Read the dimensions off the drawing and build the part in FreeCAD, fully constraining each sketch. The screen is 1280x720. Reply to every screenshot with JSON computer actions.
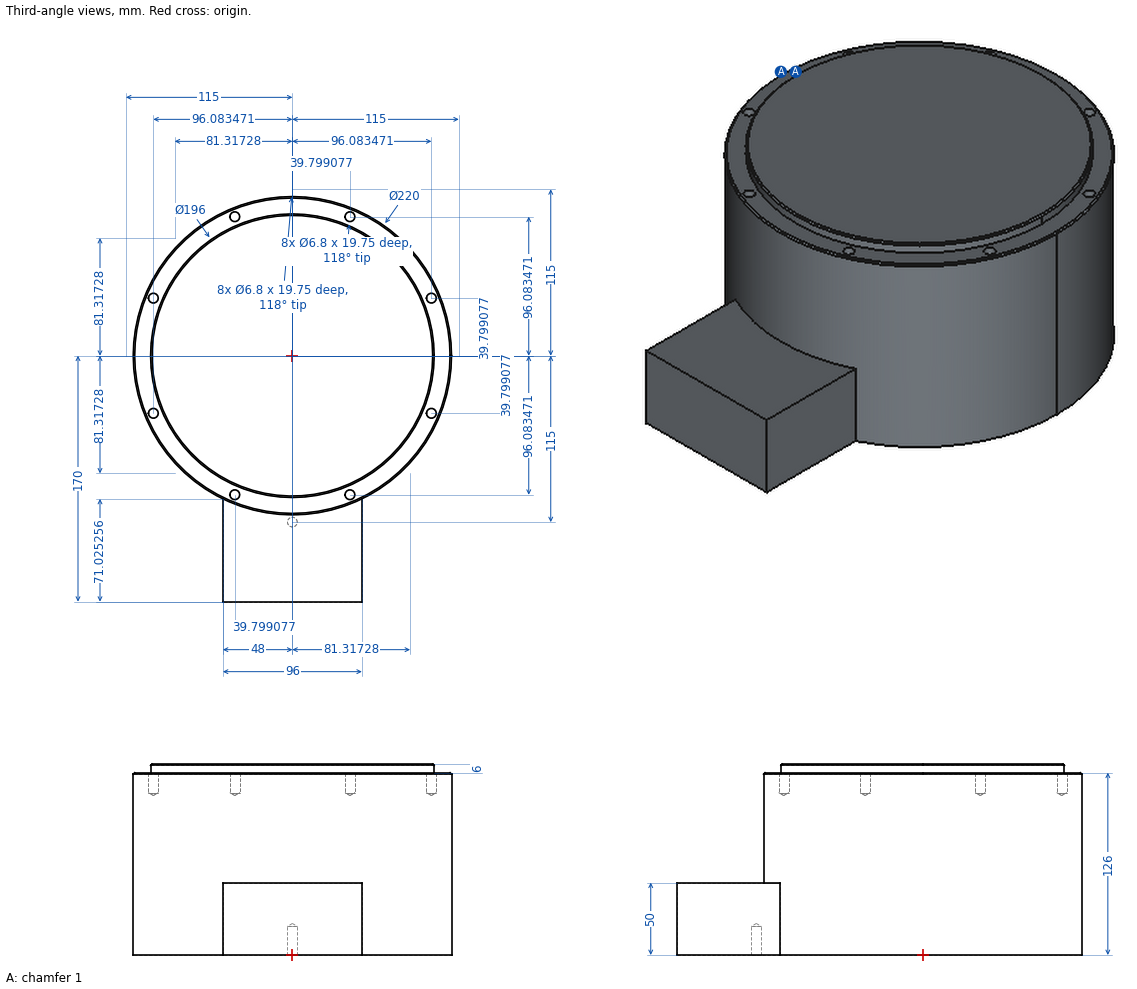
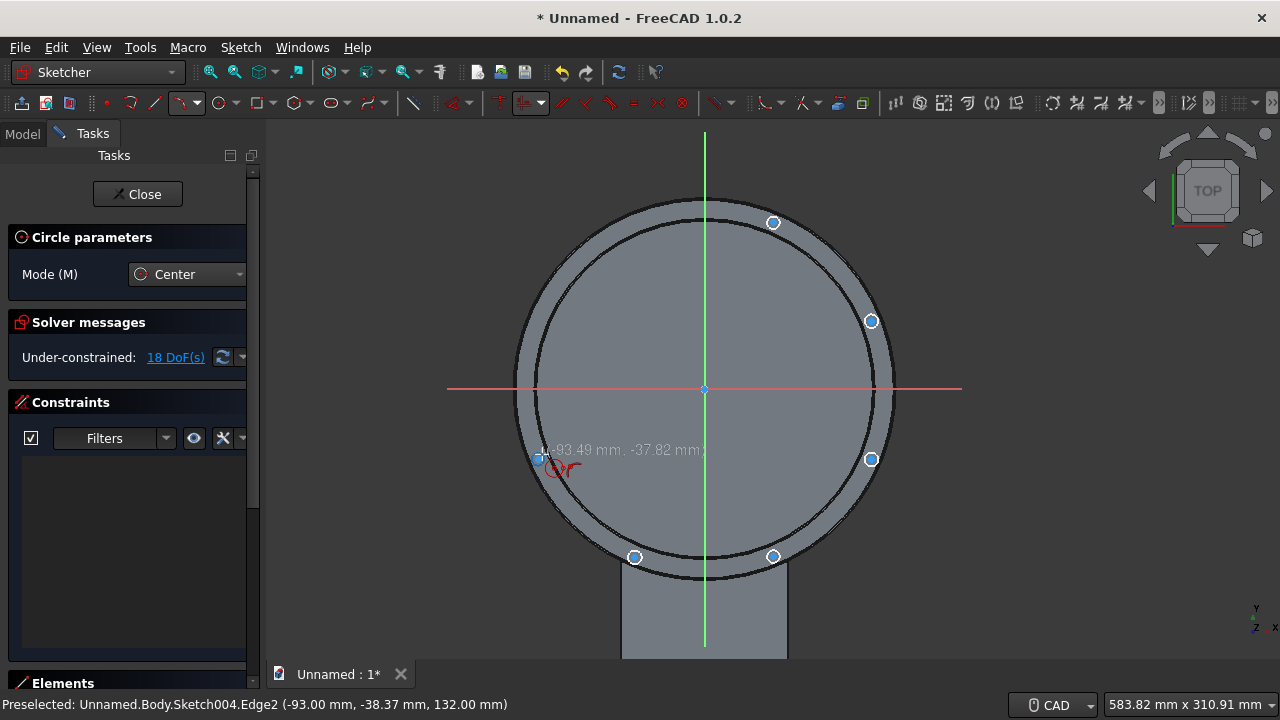
{"action": "scroll", "coordinate": [538, 320], "scroll_direction": "up", "scroll_amount": 7}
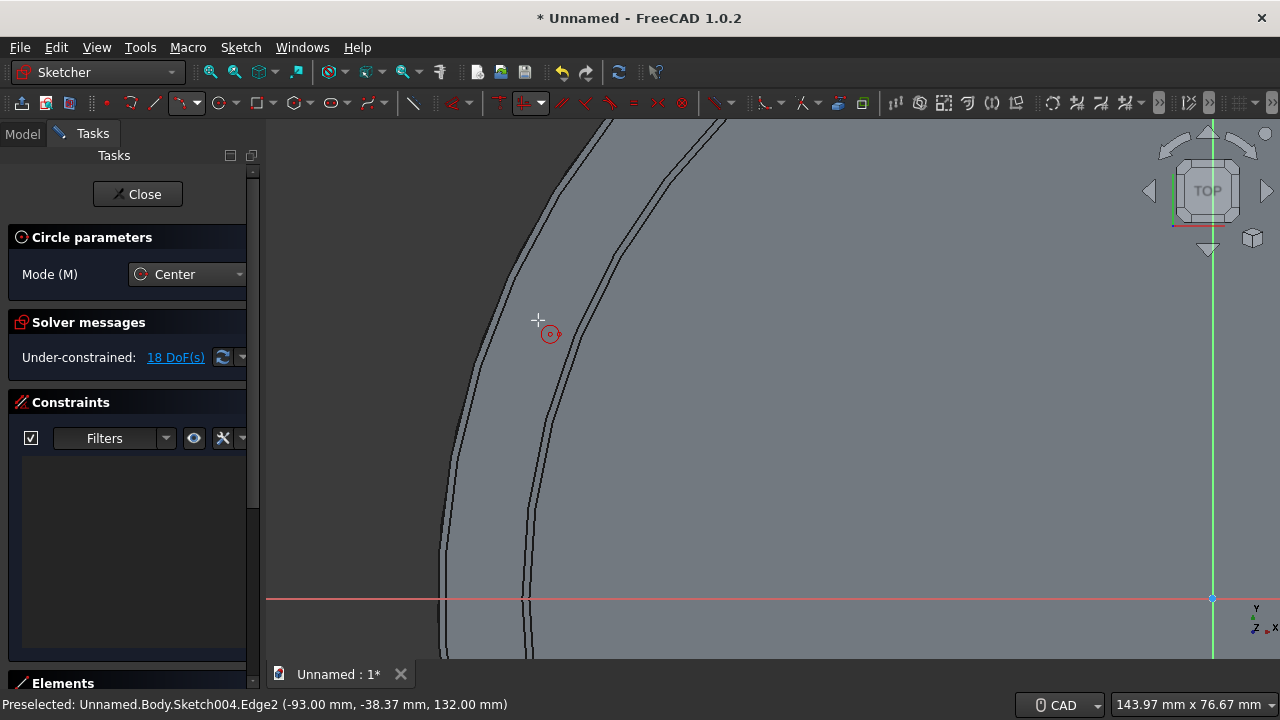
{"action": "scroll", "coordinate": [538, 320], "scroll_direction": "down", "scroll_amount": 7}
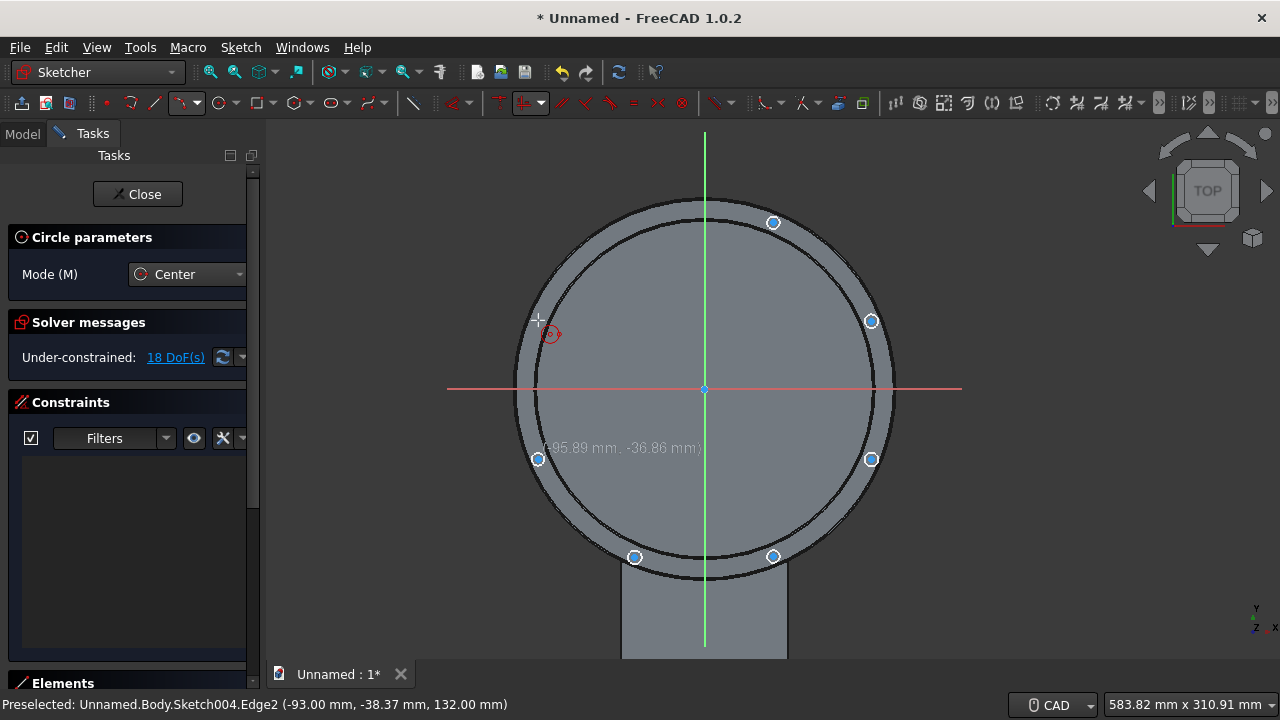
{"action": "left_click", "coordinate": [538, 320]}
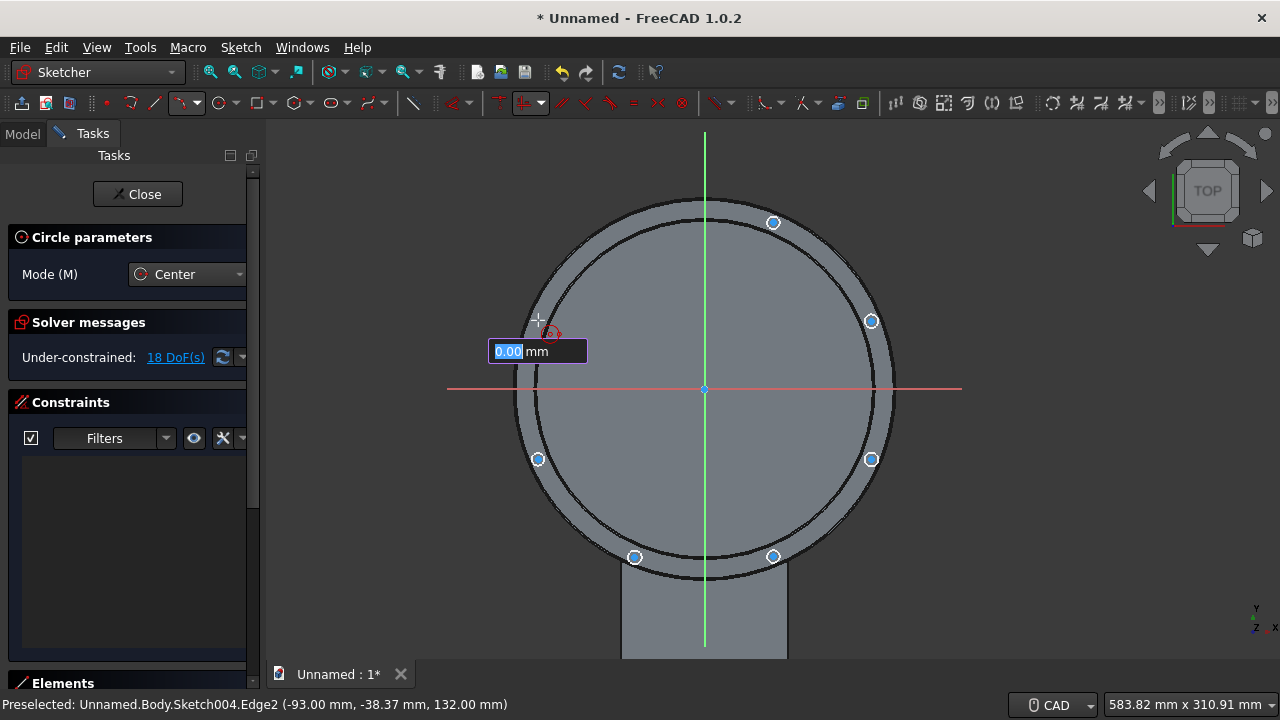
{"action": "scroll", "coordinate": [542, 316], "scroll_direction": "up", "scroll_amount": 5}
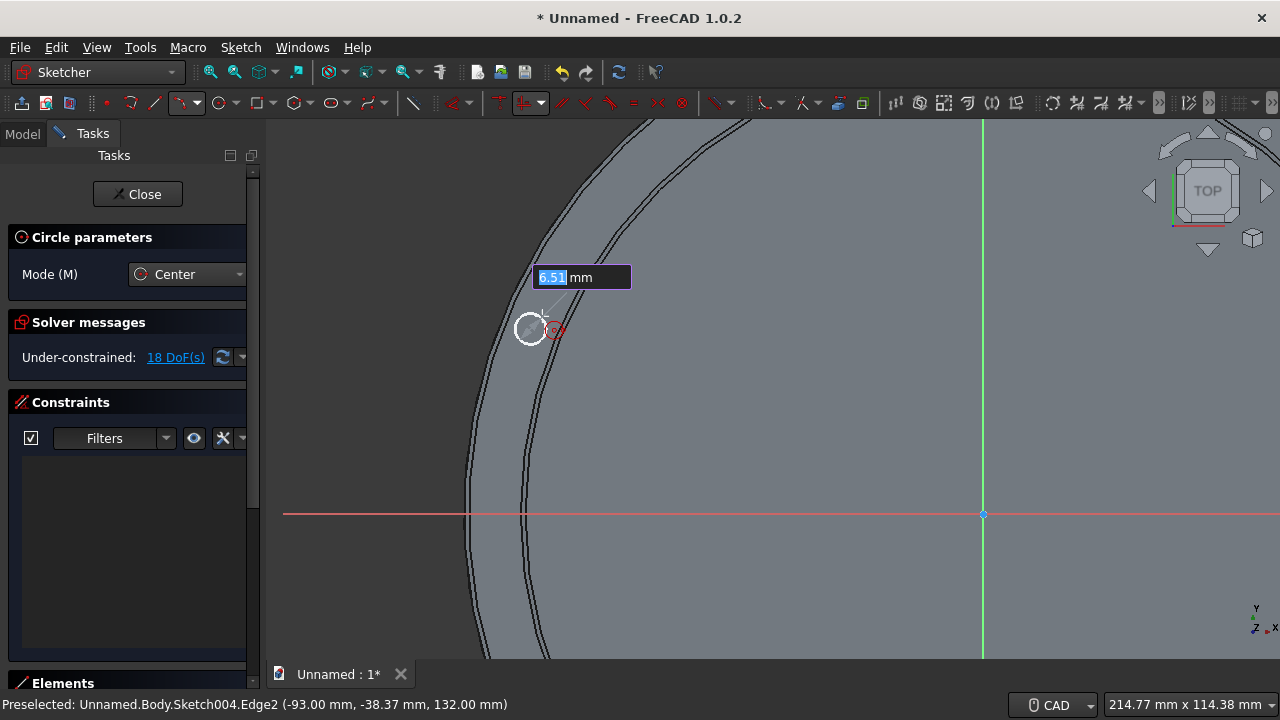
{"action": "left_click", "coordinate": [541, 315]}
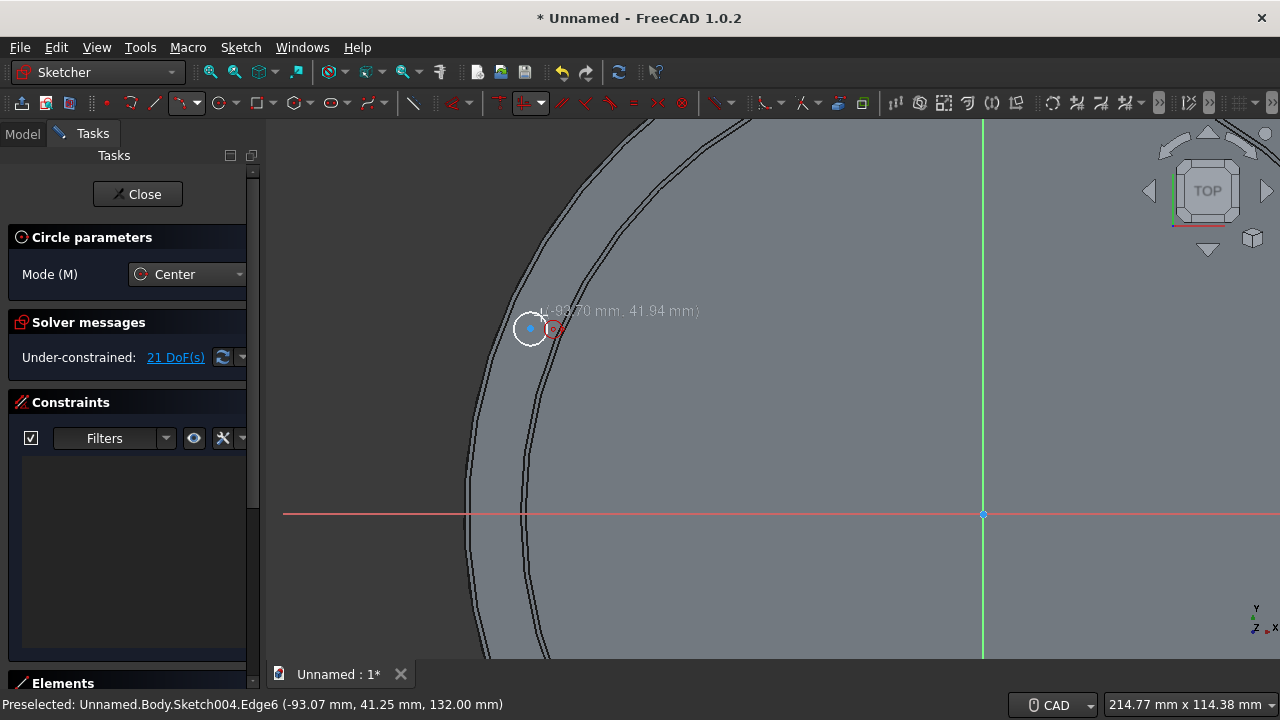
{"action": "scroll", "coordinate": [542, 316], "scroll_direction": "down", "scroll_amount": 5}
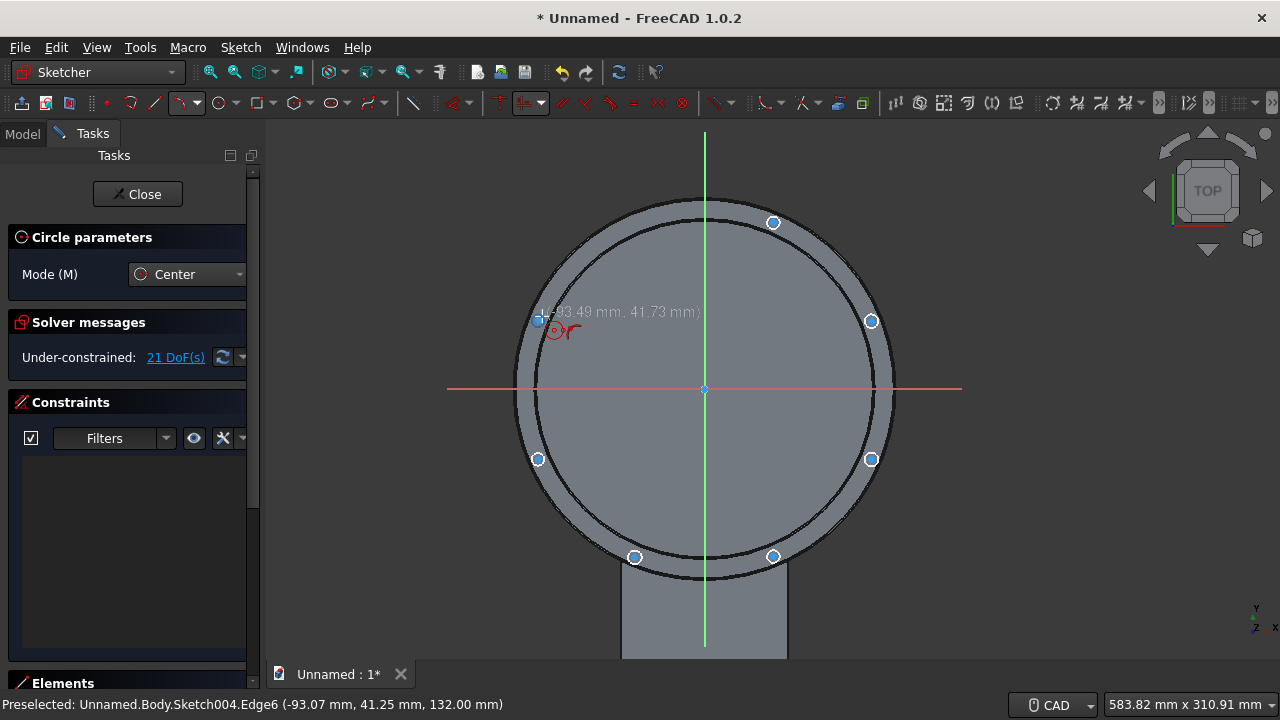
{"action": "scroll", "coordinate": [635, 222], "scroll_direction": "up", "scroll_amount": 7}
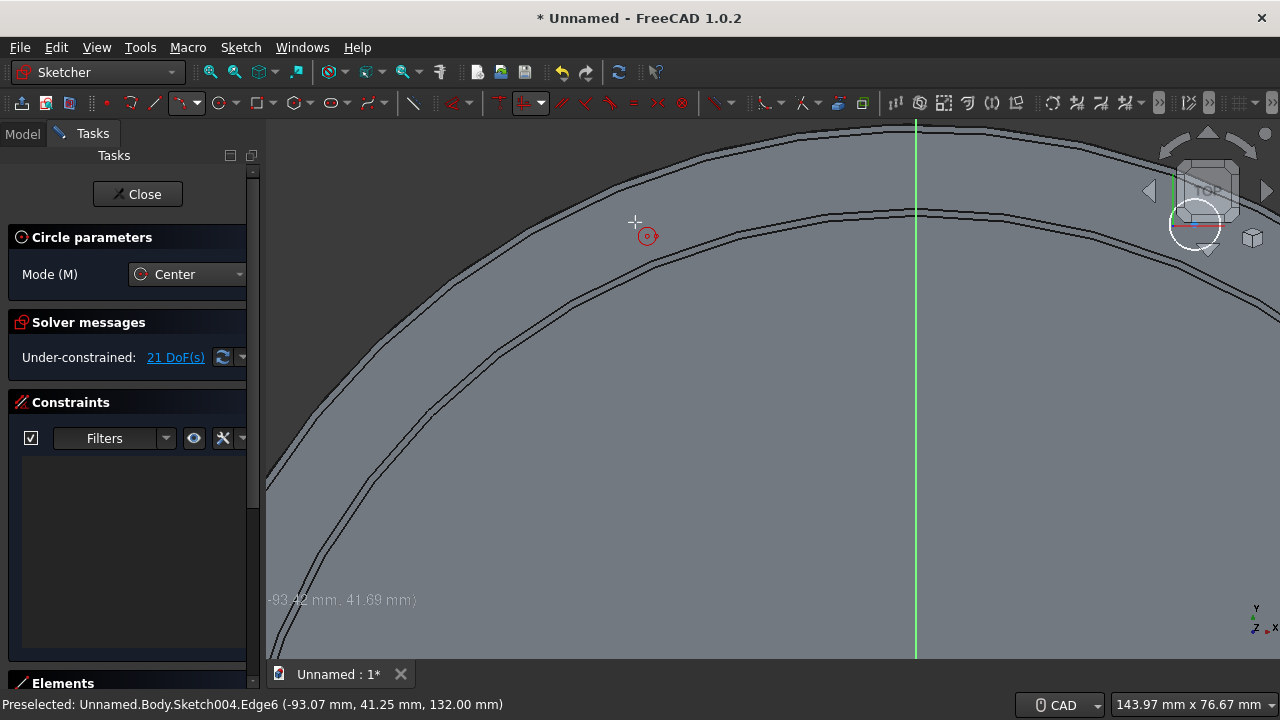
{"action": "scroll", "coordinate": [635, 222], "scroll_direction": "down", "scroll_amount": 7}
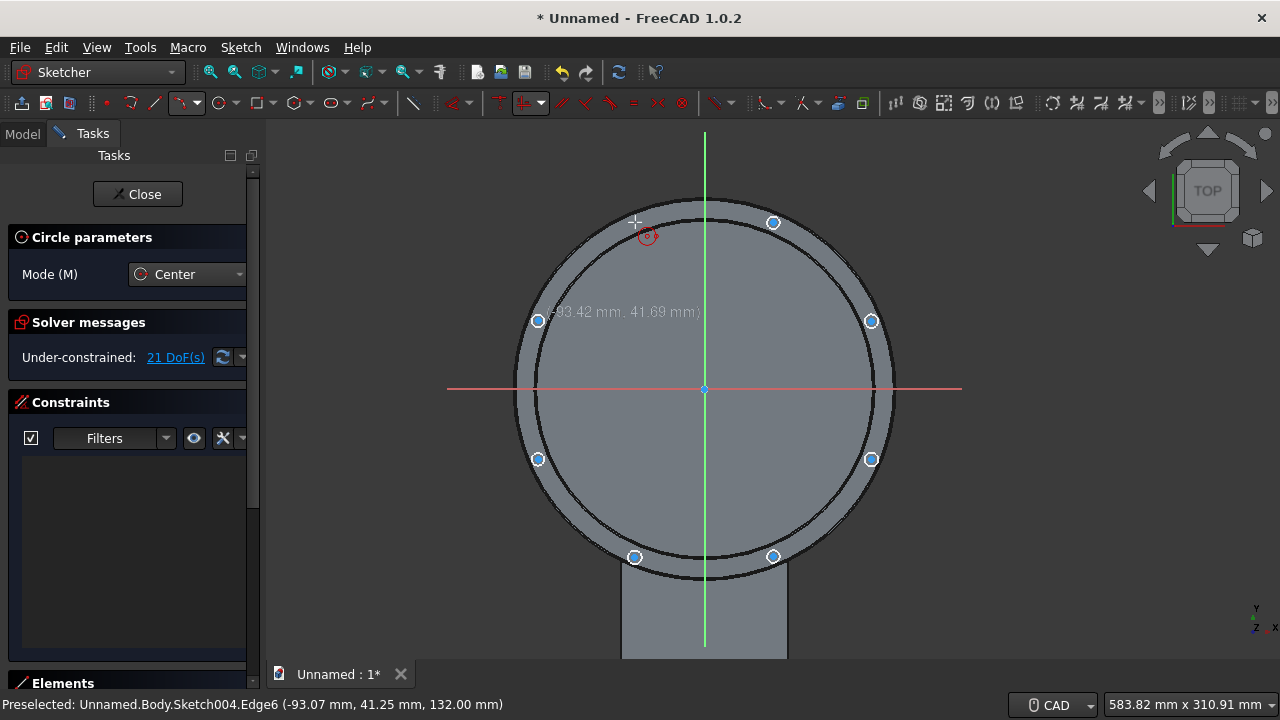
{"action": "left_click", "coordinate": [635, 222]}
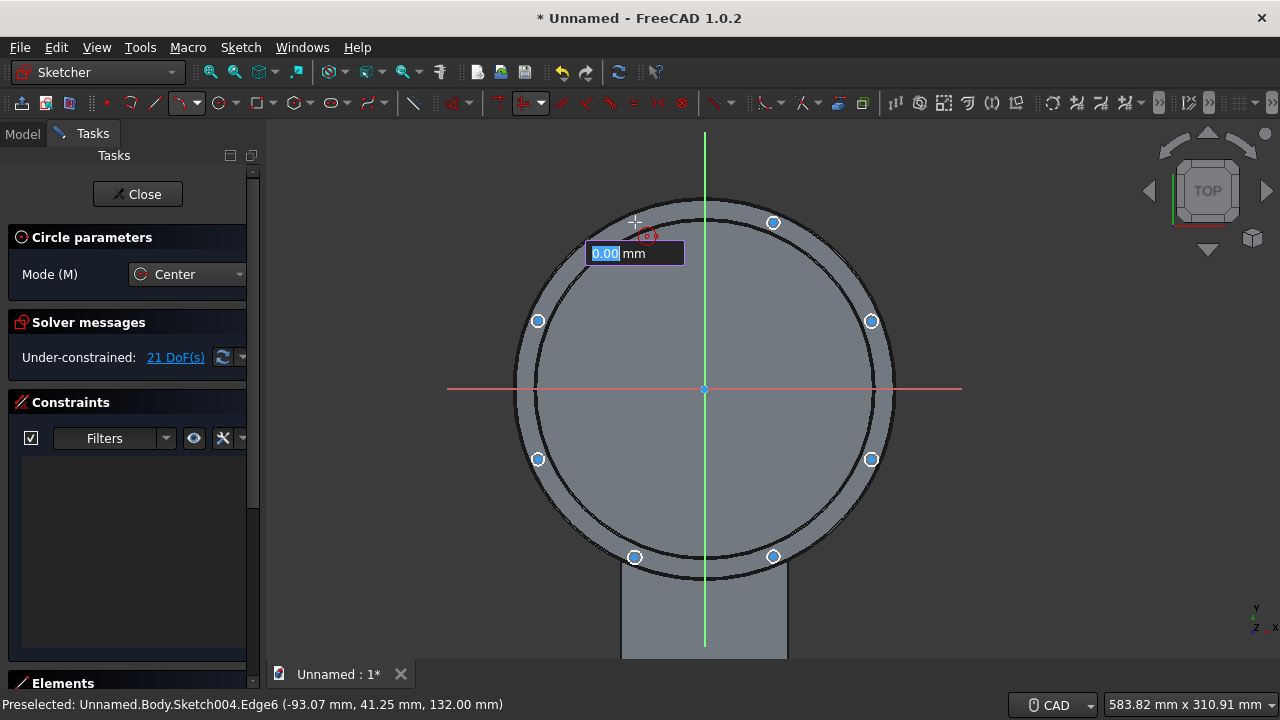
{"action": "scroll", "coordinate": [640, 218], "scroll_direction": "up", "scroll_amount": 5}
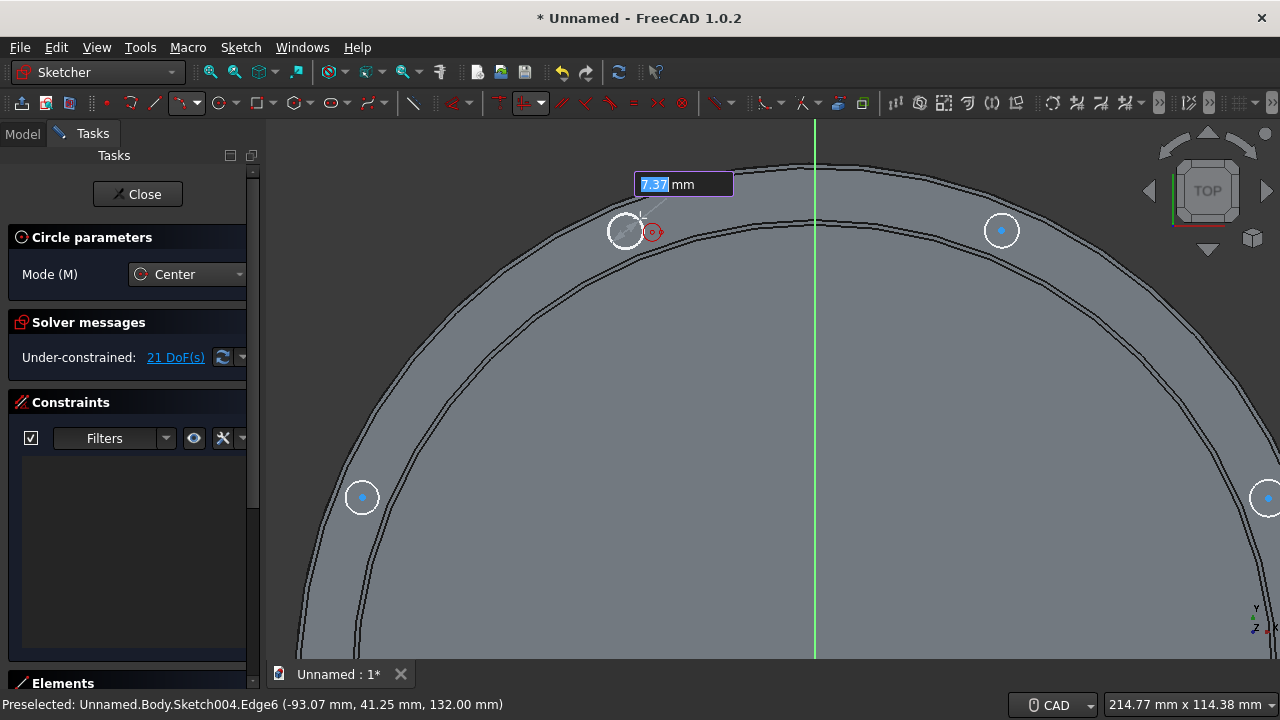
{"action": "left_click", "coordinate": [638, 218]}
{"action": "key", "text": "Escape"}